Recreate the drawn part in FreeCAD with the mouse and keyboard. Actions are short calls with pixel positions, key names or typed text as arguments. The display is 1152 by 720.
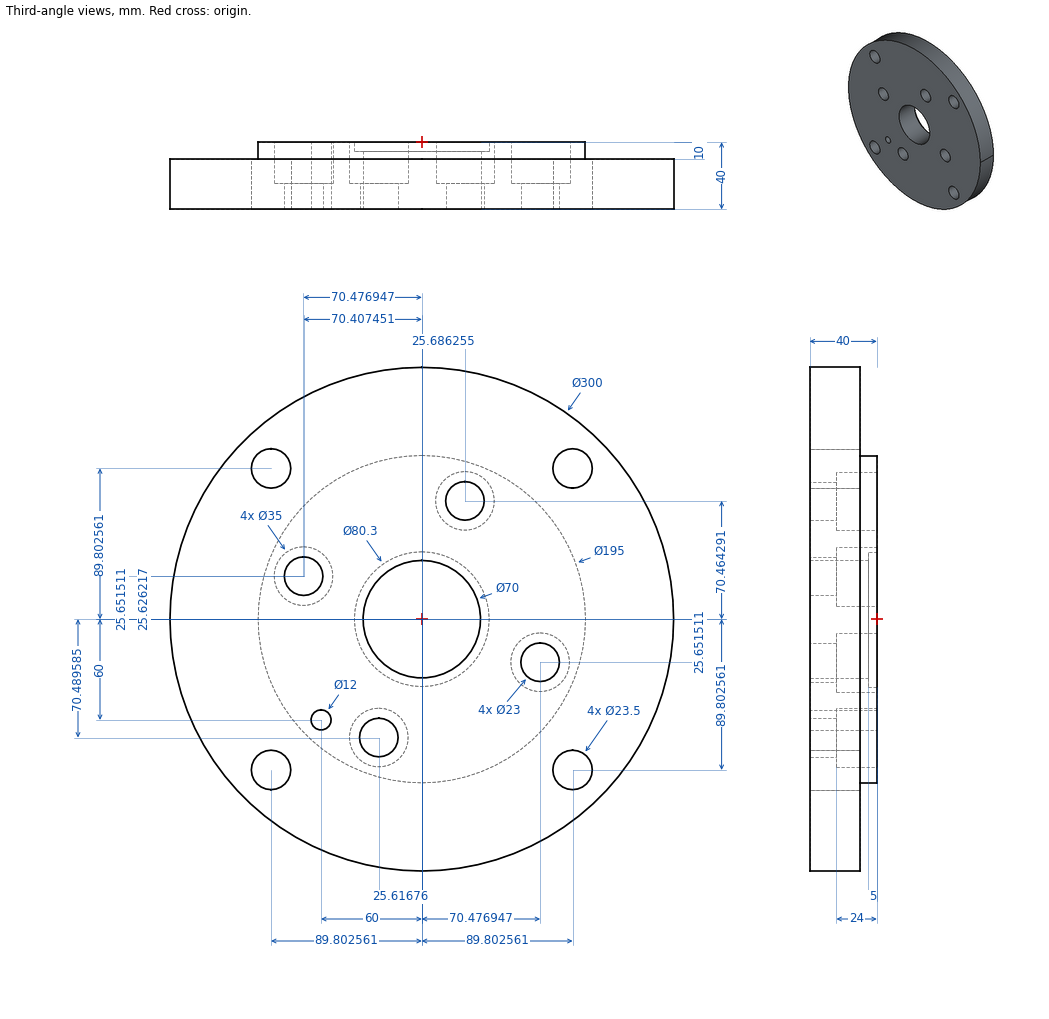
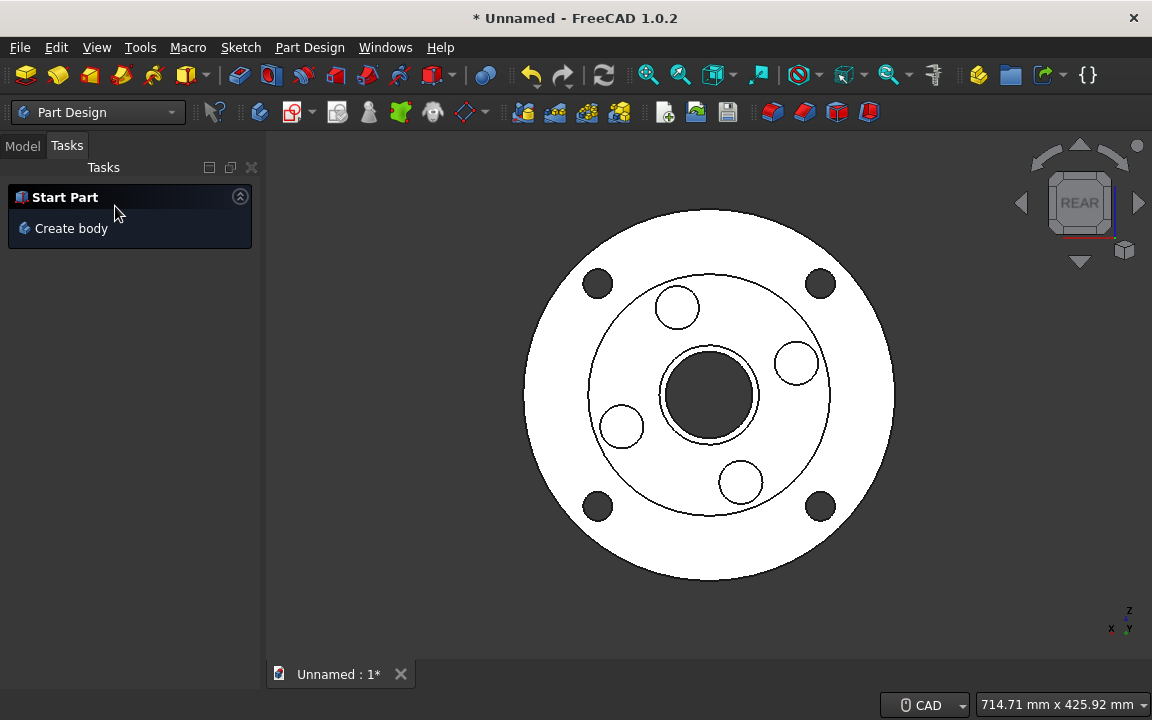
click(640, 359)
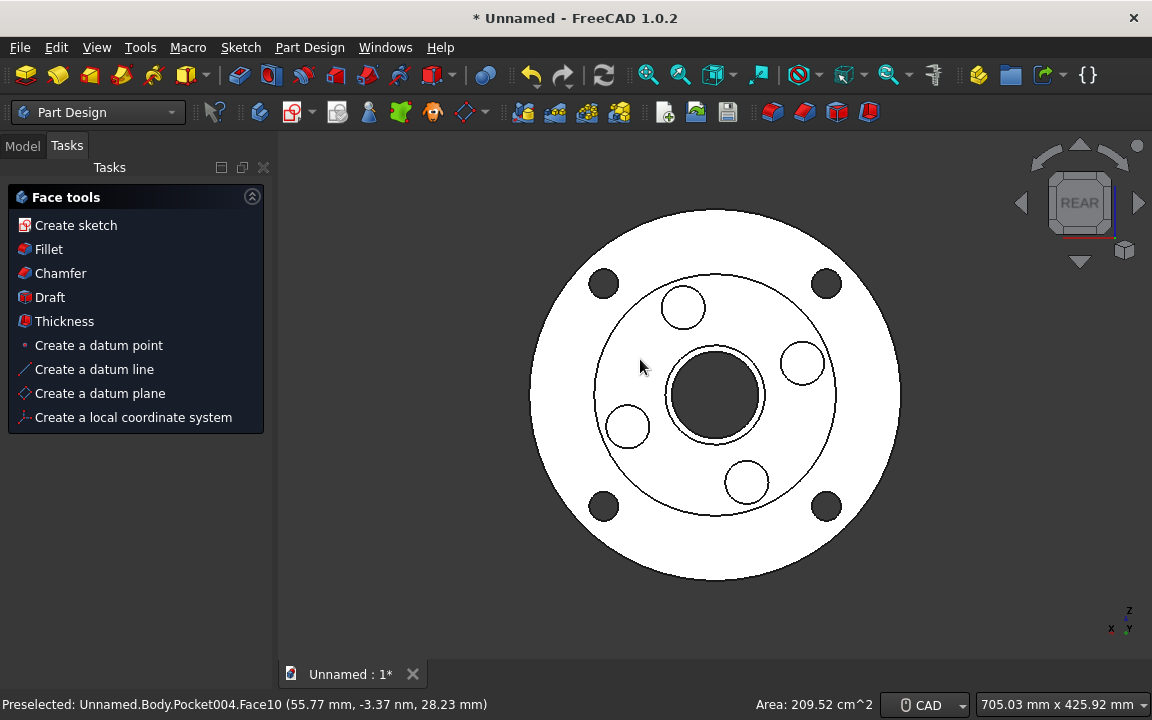
click(292, 112)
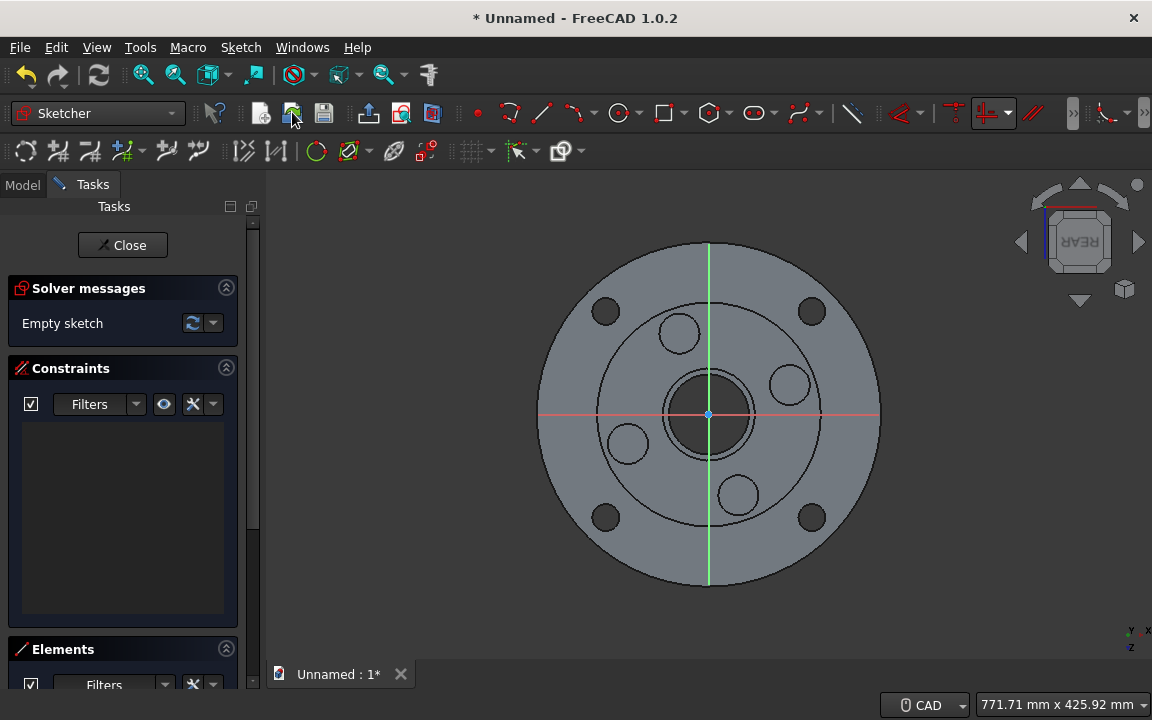
scroll(848, 414, up, 2)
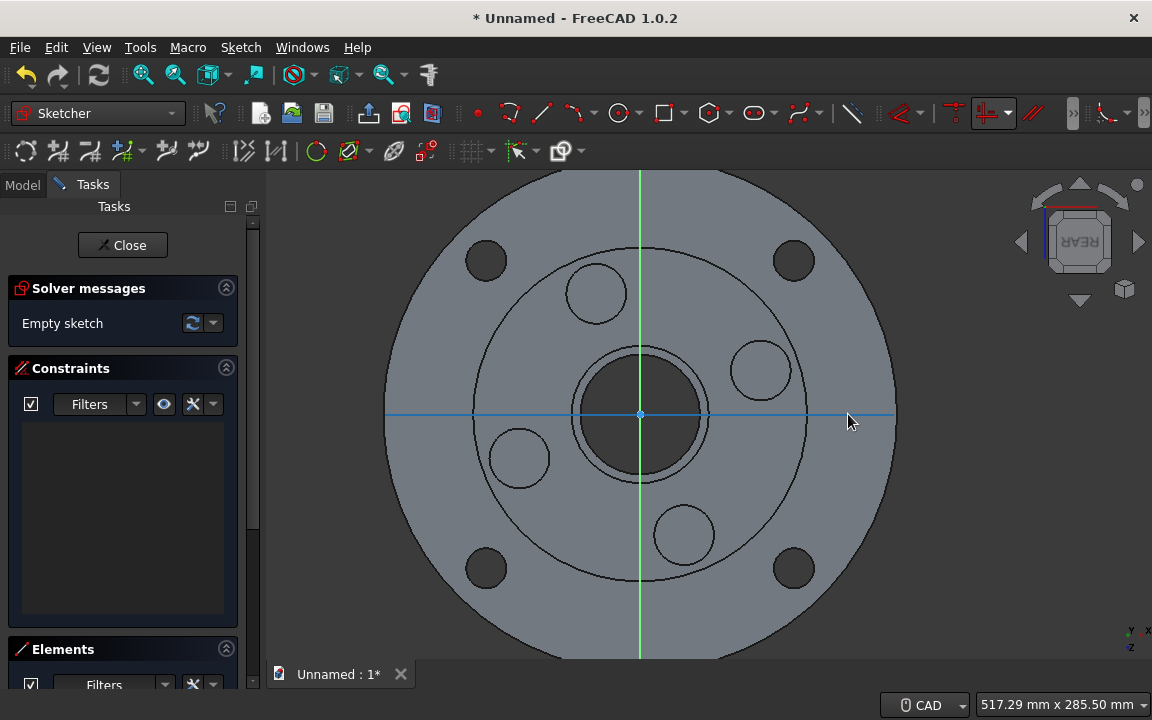
click(620, 114)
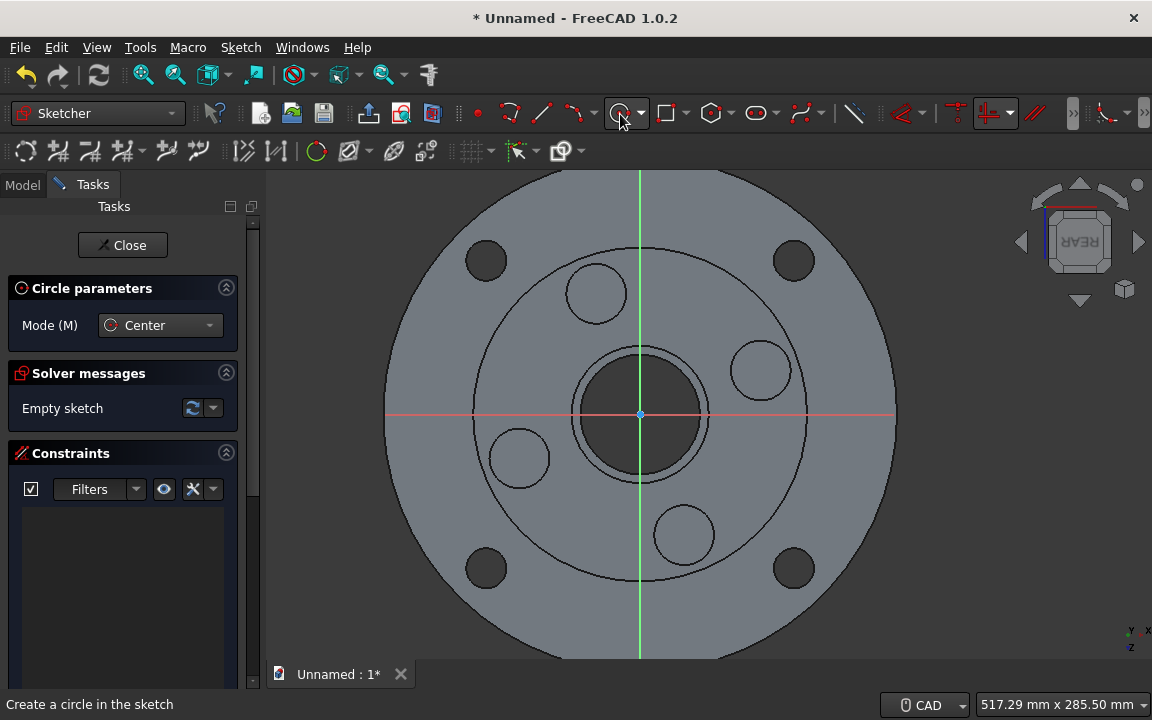
click(761, 371)
move(775, 357)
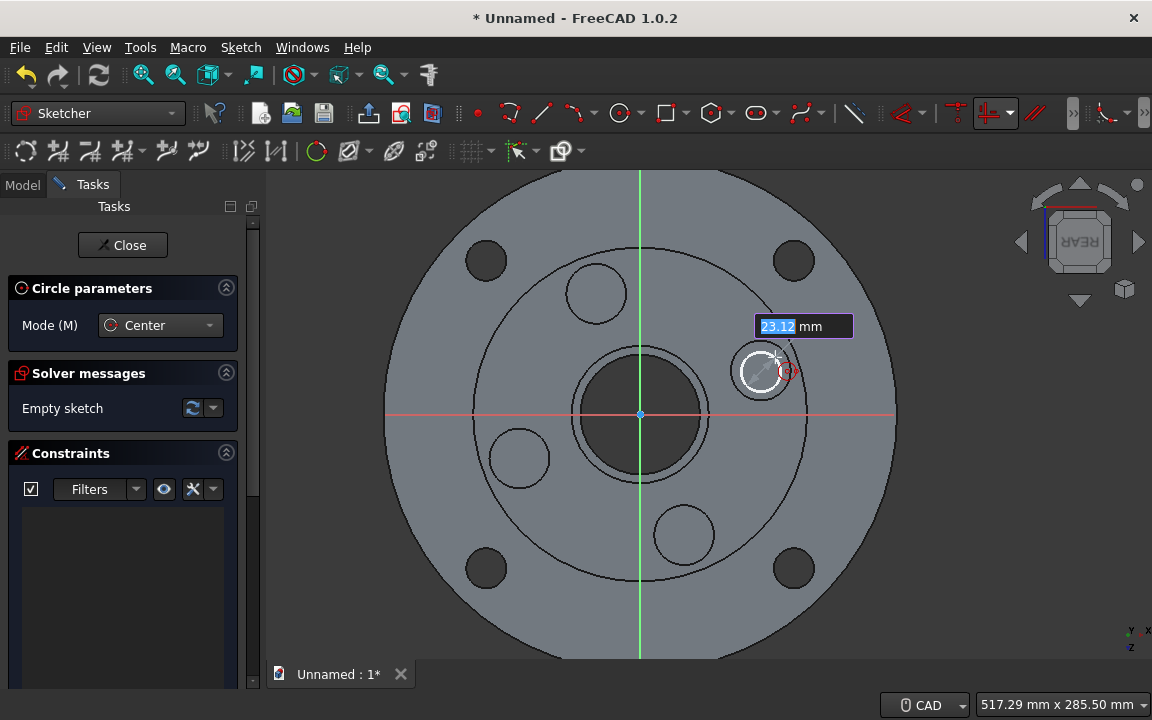
text(23)
key(Return)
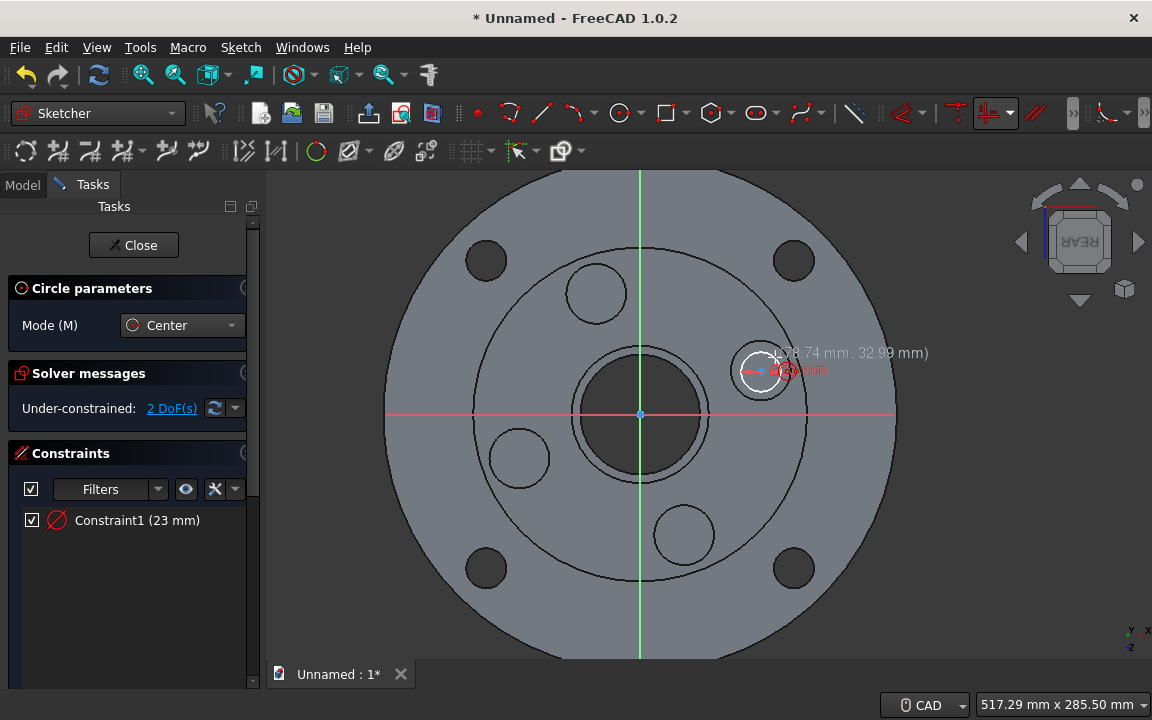
click(520, 458)
move(533, 444)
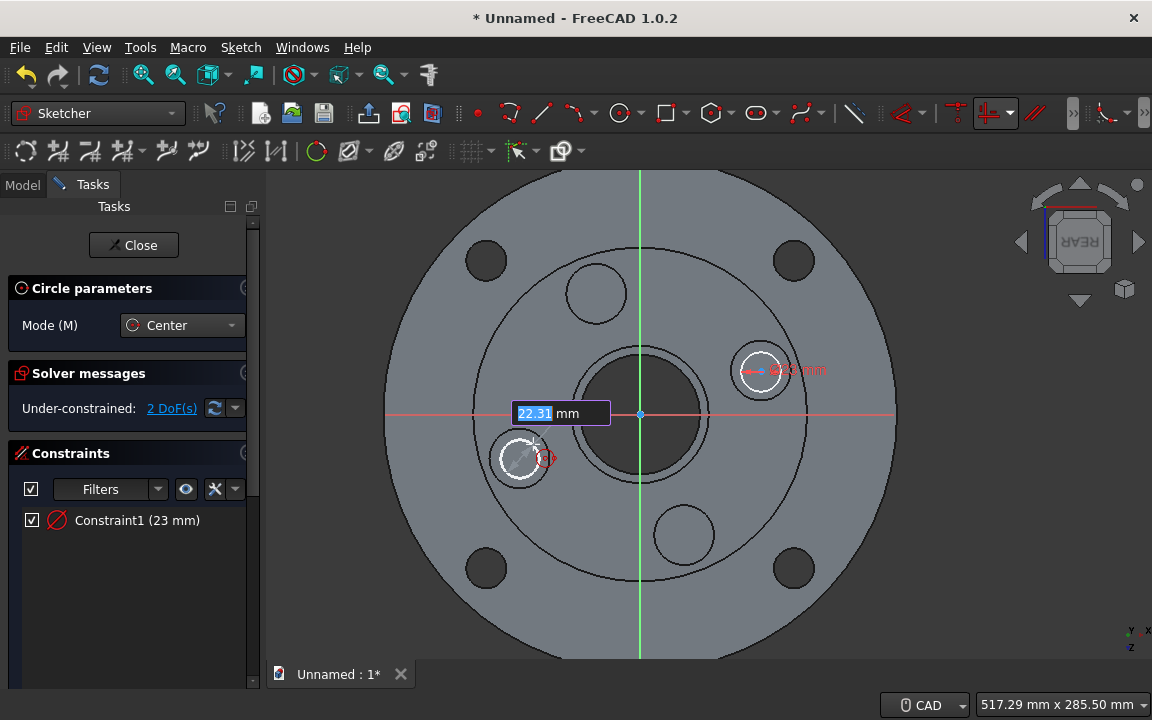
text(23)
key(Return)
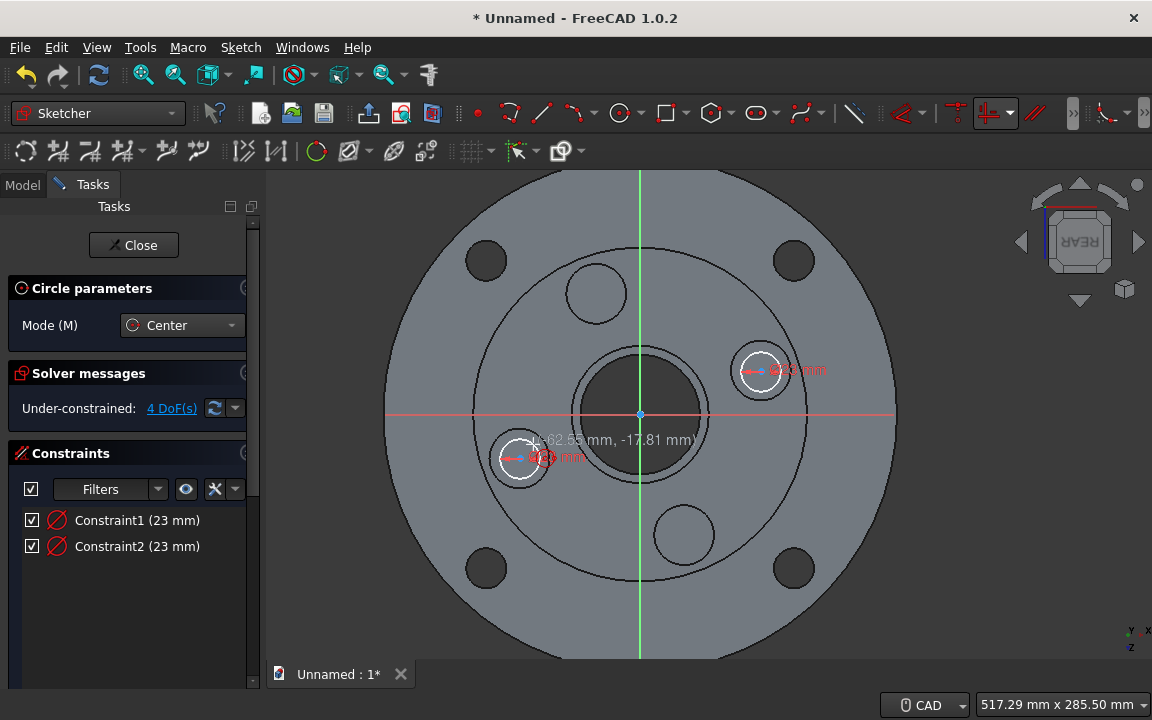
click(596, 294)
move(610, 280)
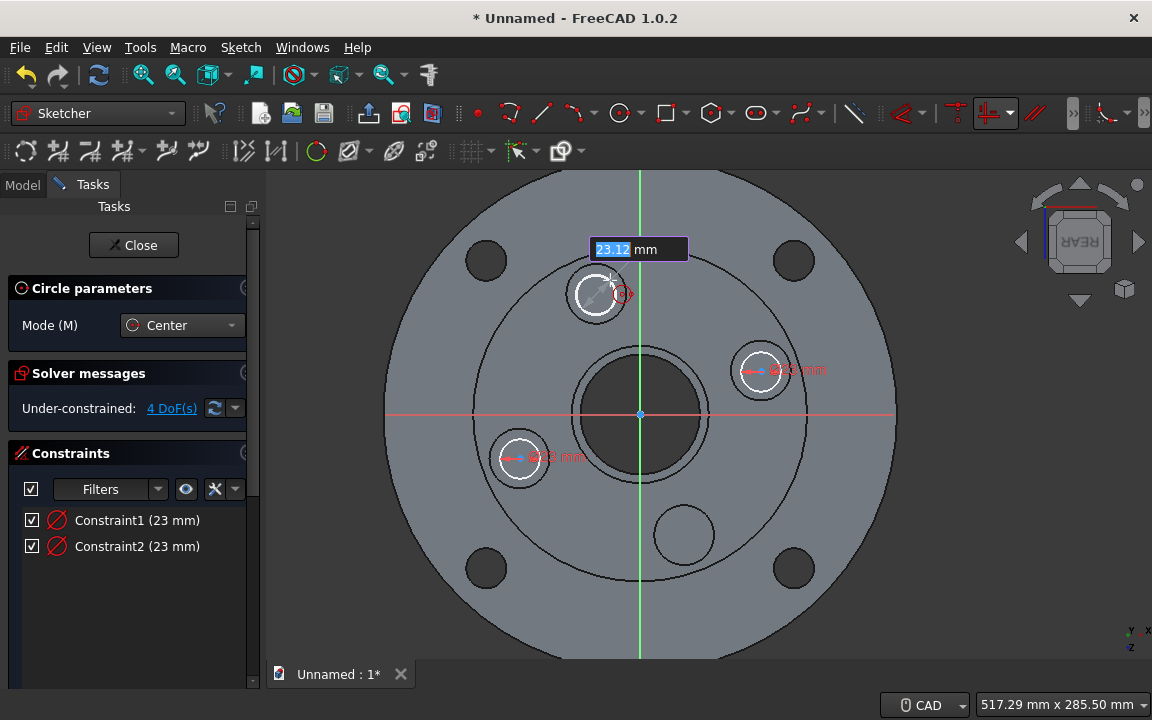
text(23)
key(Return)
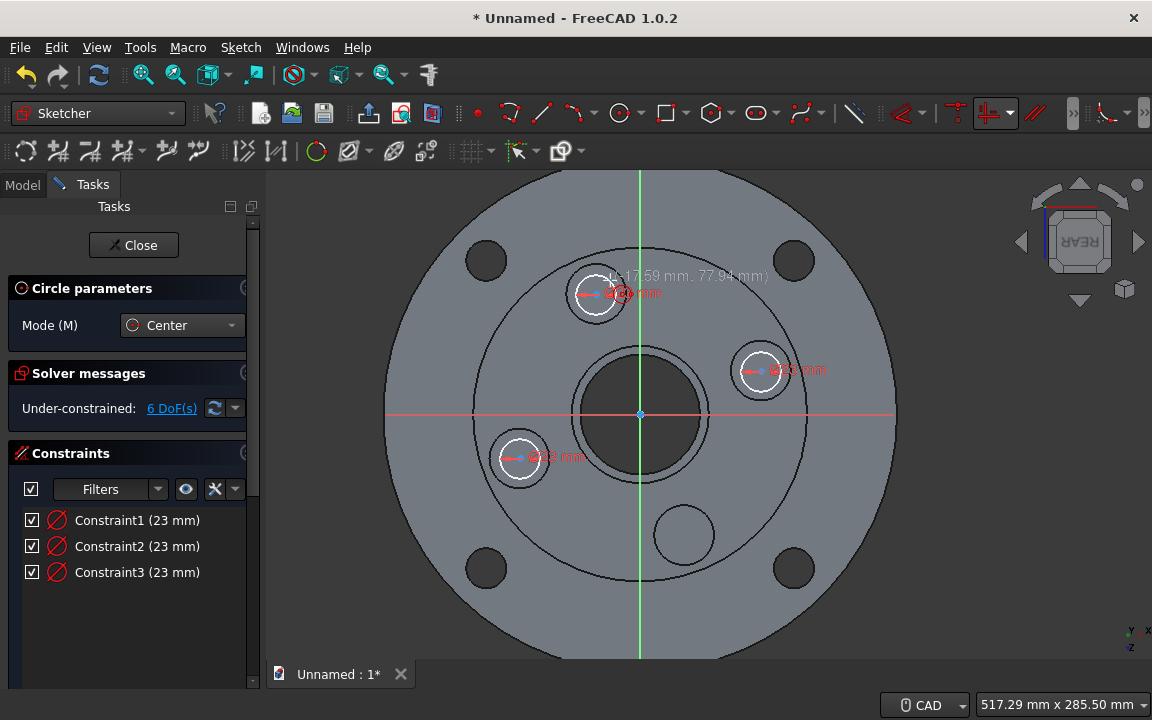
click(684, 535)
move(698, 521)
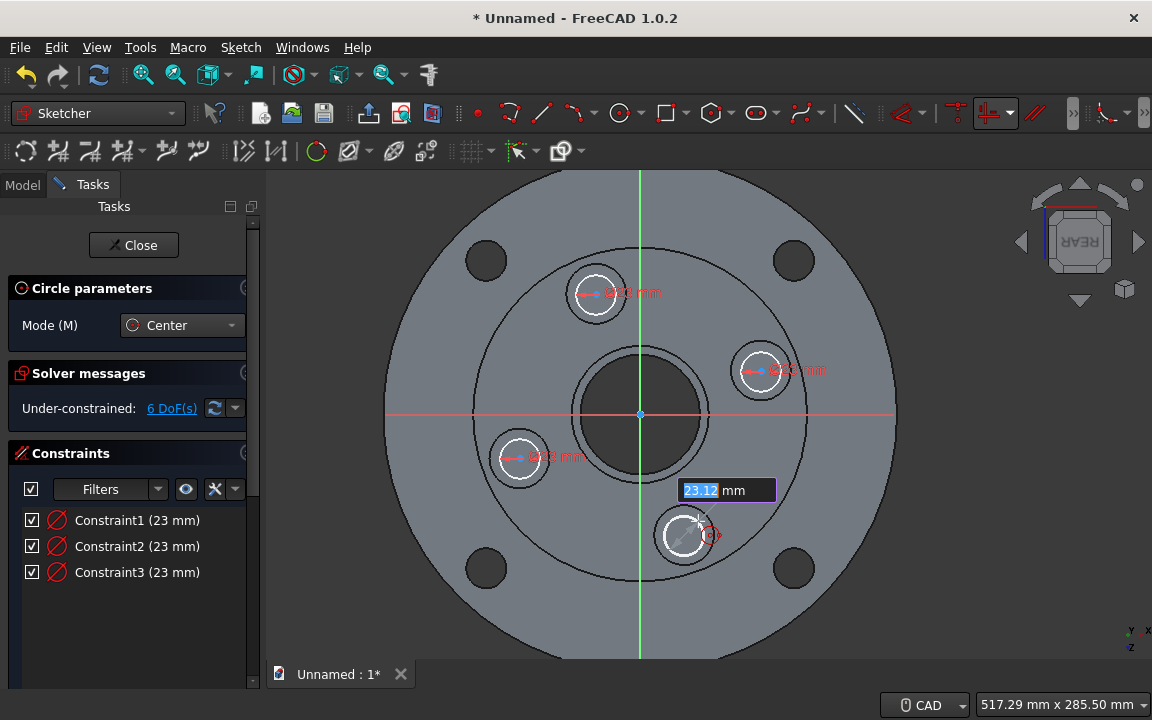
text(23)
key(Return)
key(Escape)